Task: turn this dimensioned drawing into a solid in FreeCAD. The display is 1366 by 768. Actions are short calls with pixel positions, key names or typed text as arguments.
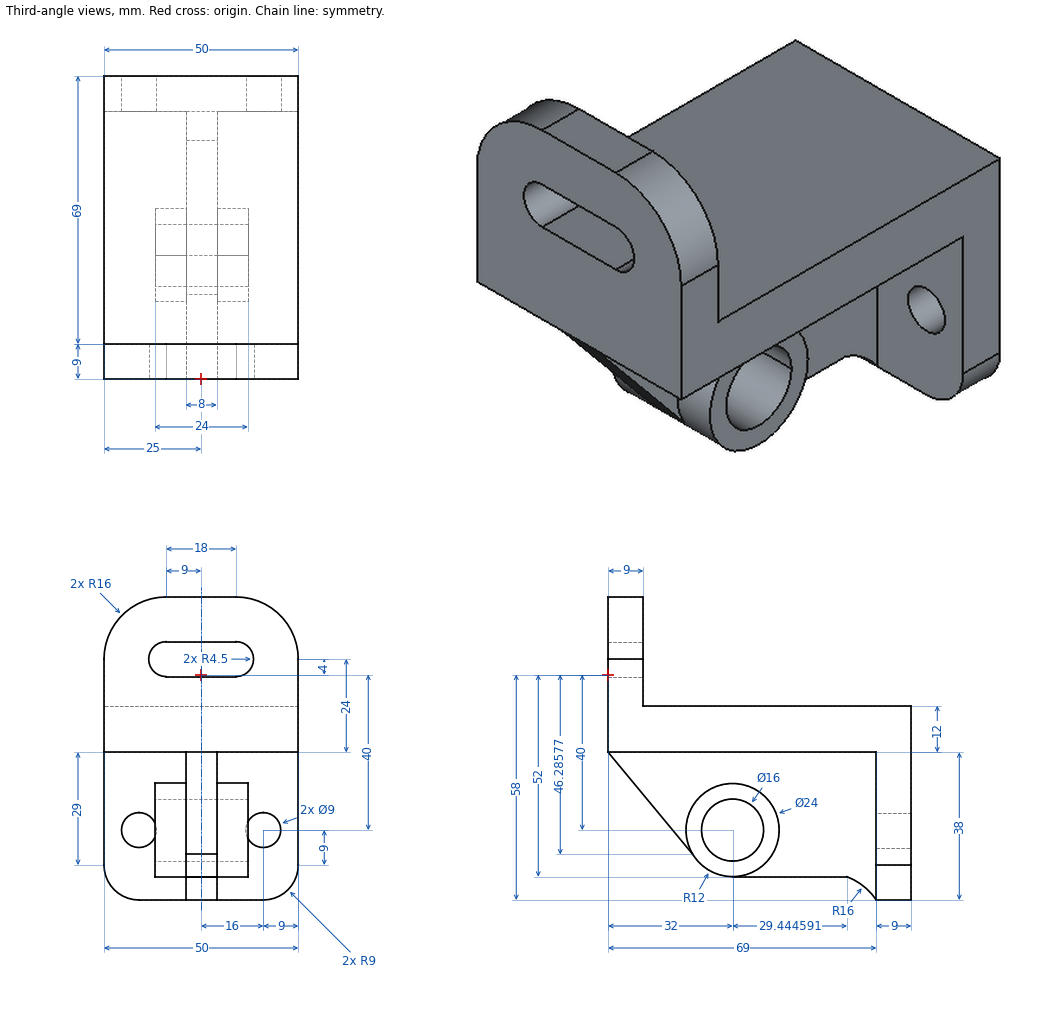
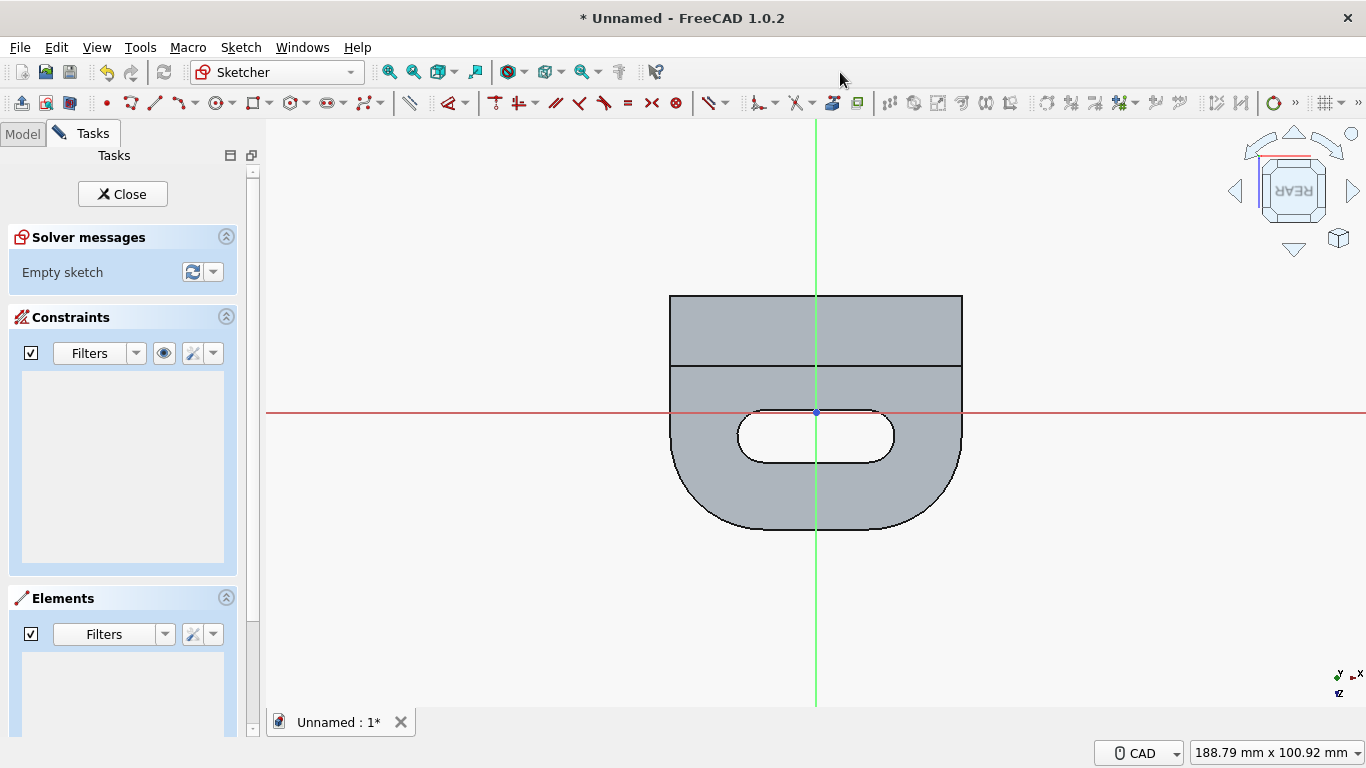
scroll(438, 679, down, 1)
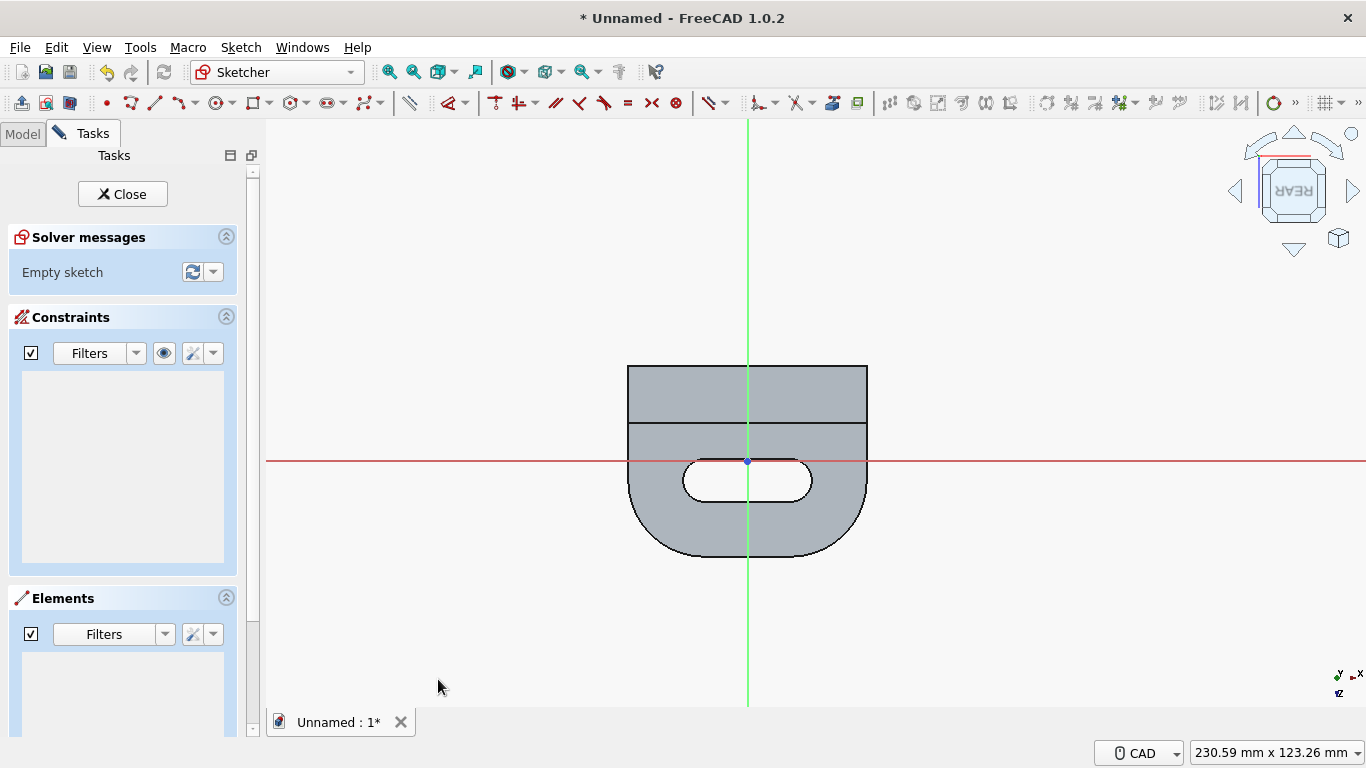
scroll(748, 147, up, 2)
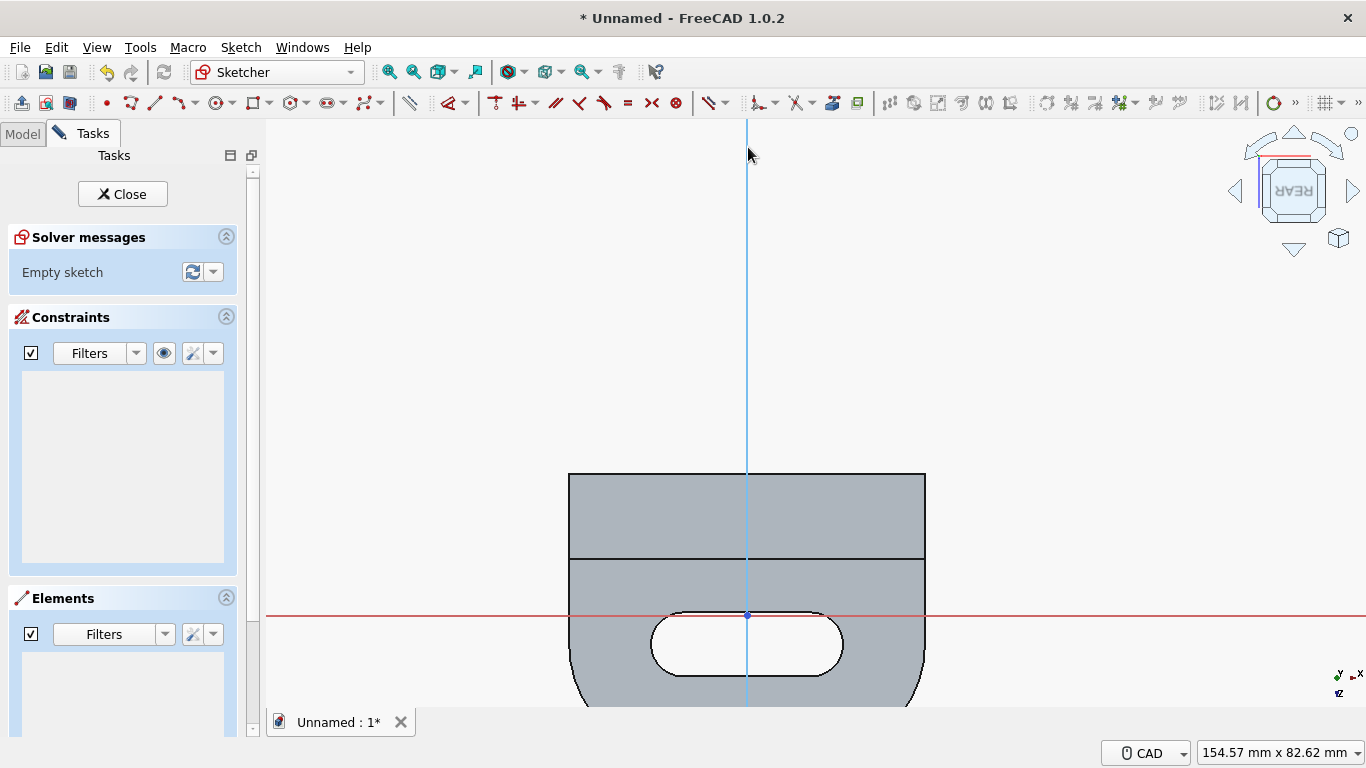
click(132, 104)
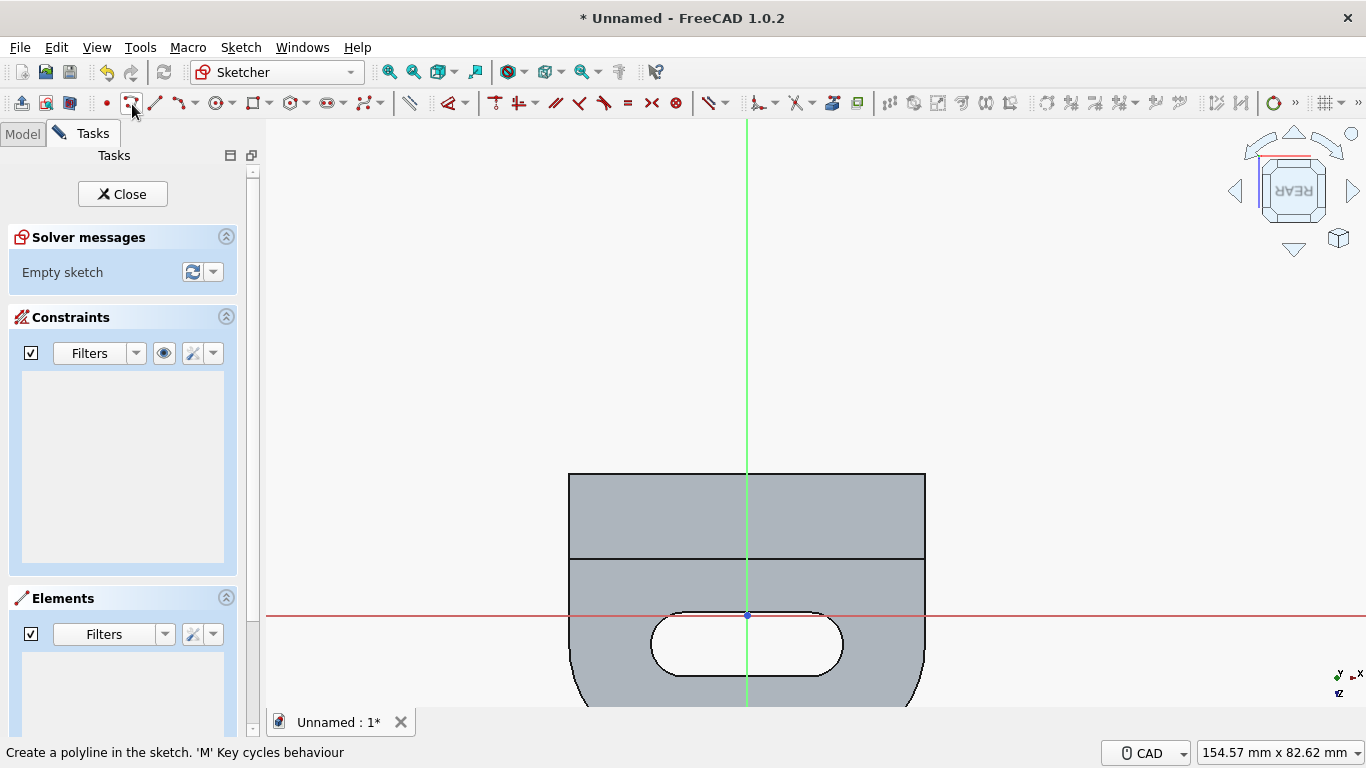
click(569, 267)
click(569, 474)
click(925, 474)
click(925, 267)
right_click(925, 267)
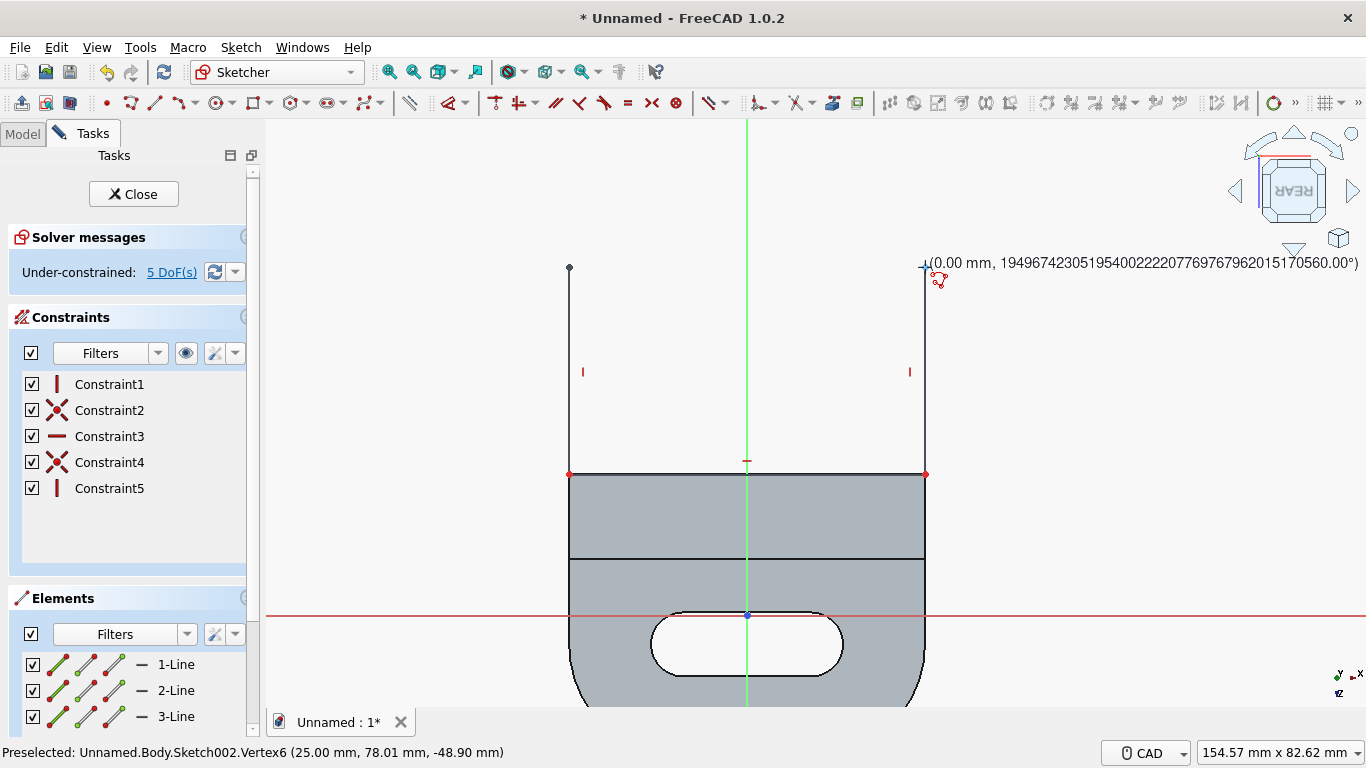
key(g)
key(l)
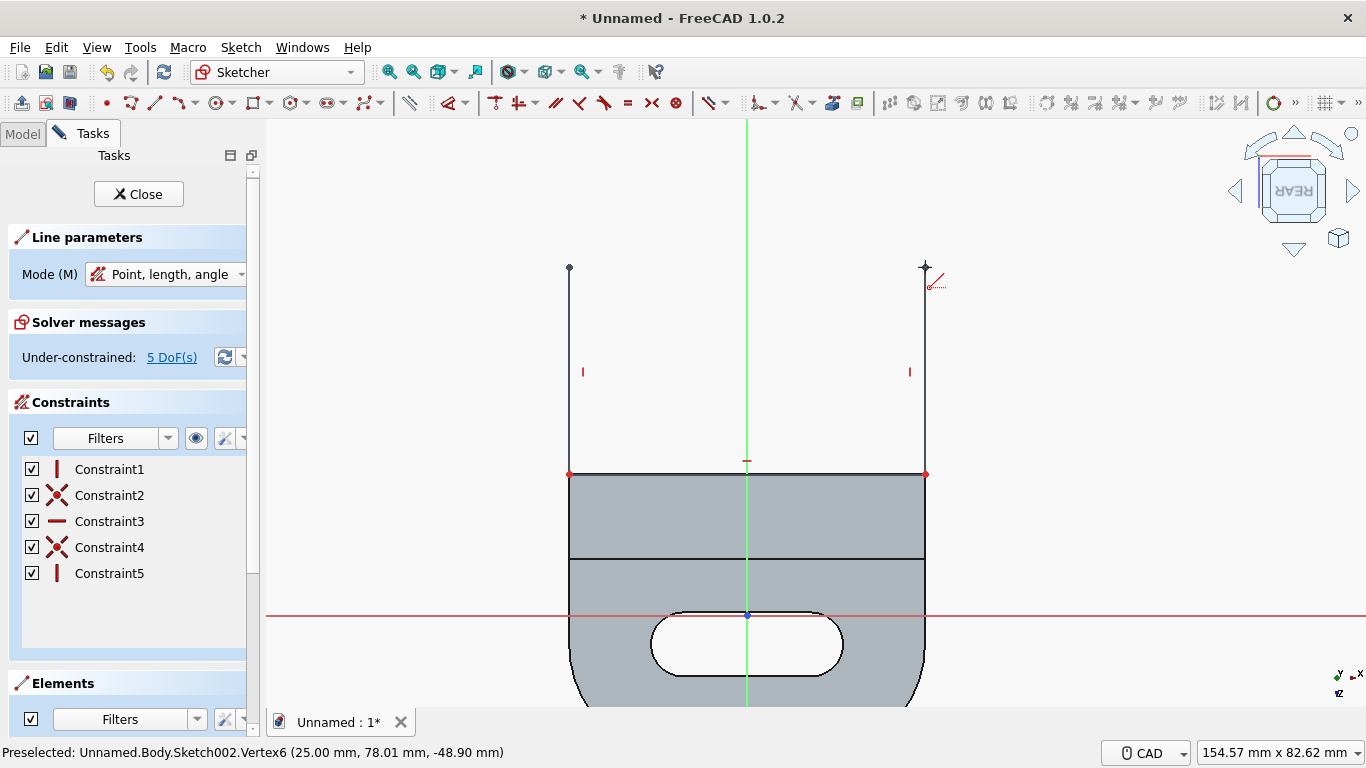
click(861, 203)
click(633, 203)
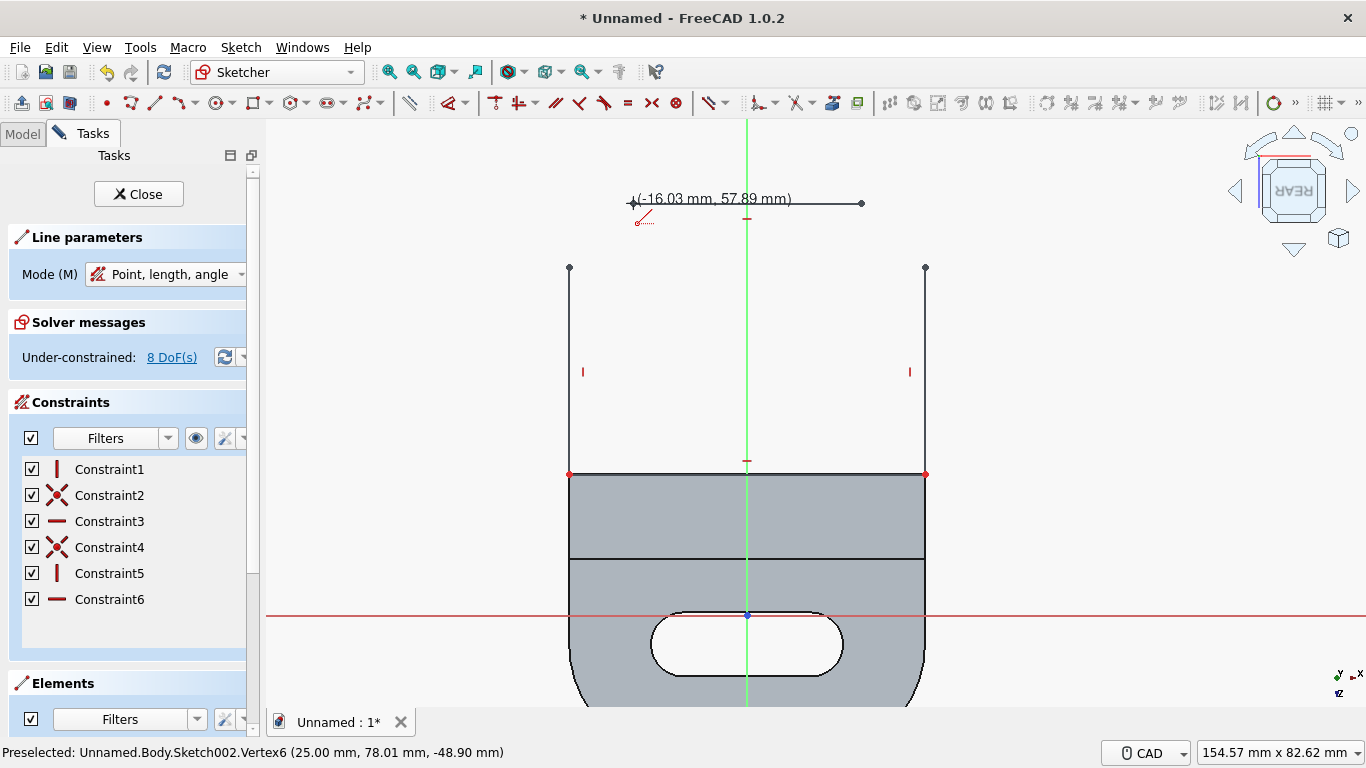
click(180, 104)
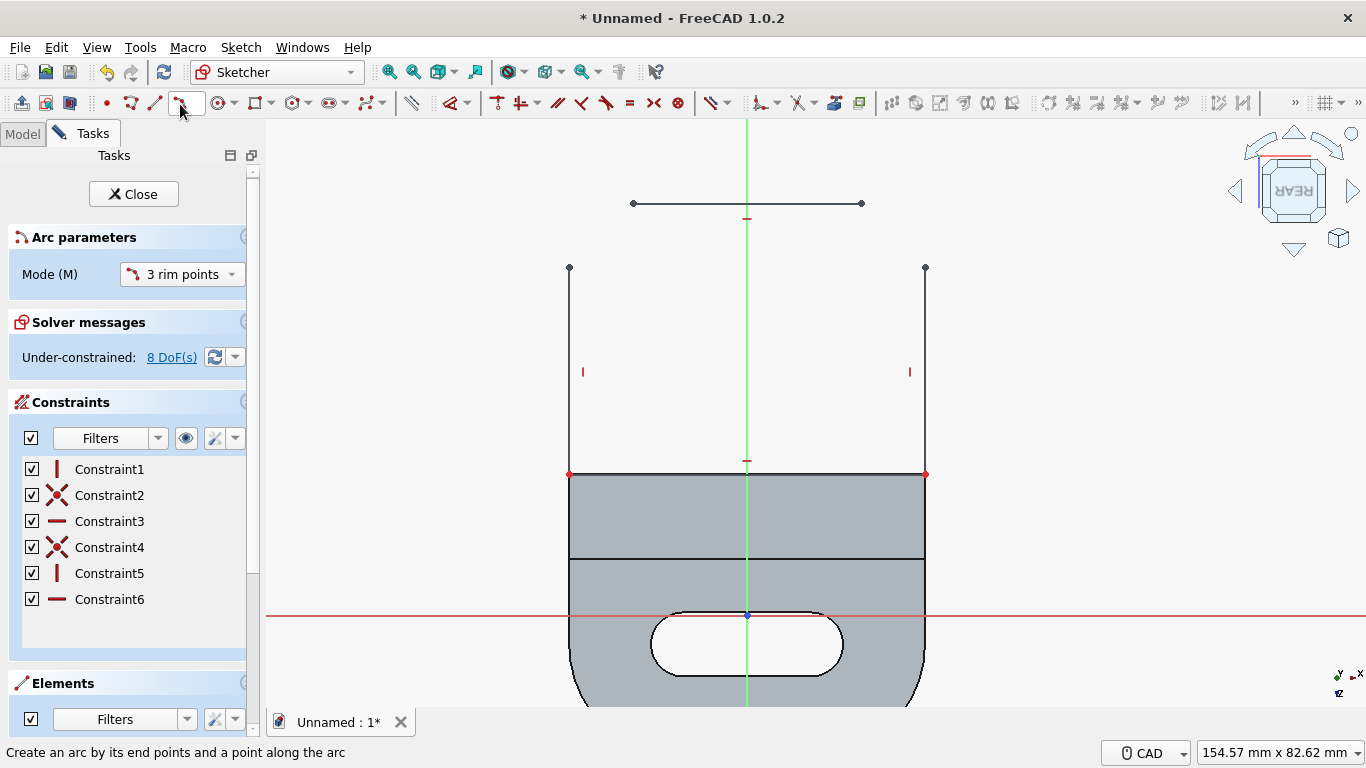
click(925, 268)
click(861, 204)
click(906, 222)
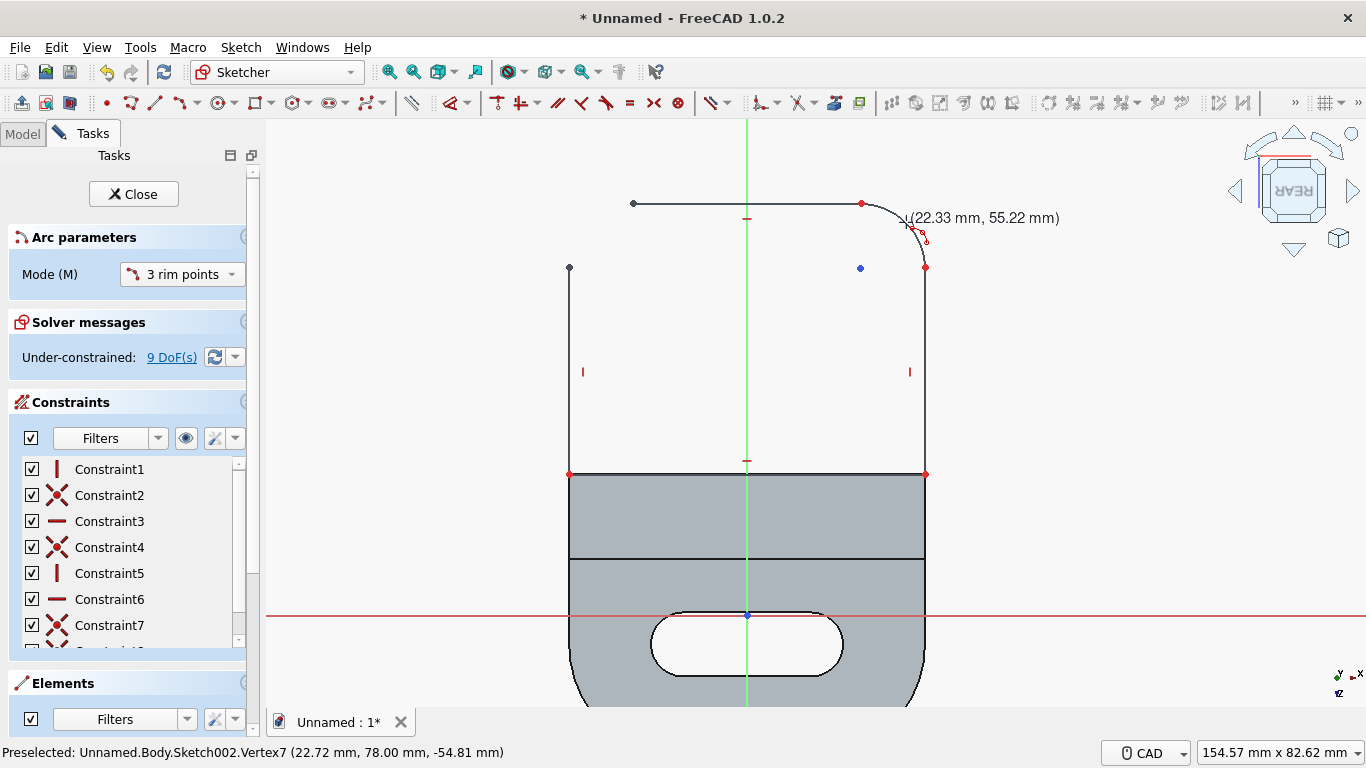
click(633, 204)
click(569, 268)
click(588, 222)